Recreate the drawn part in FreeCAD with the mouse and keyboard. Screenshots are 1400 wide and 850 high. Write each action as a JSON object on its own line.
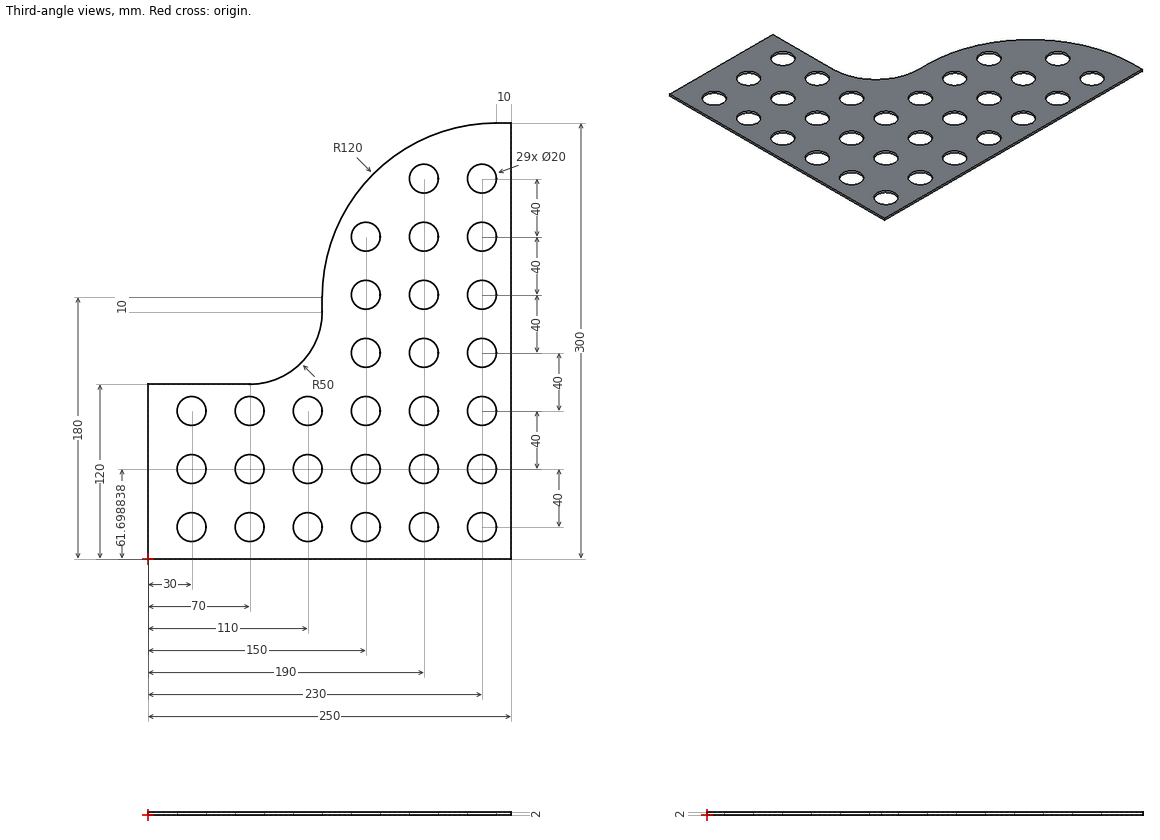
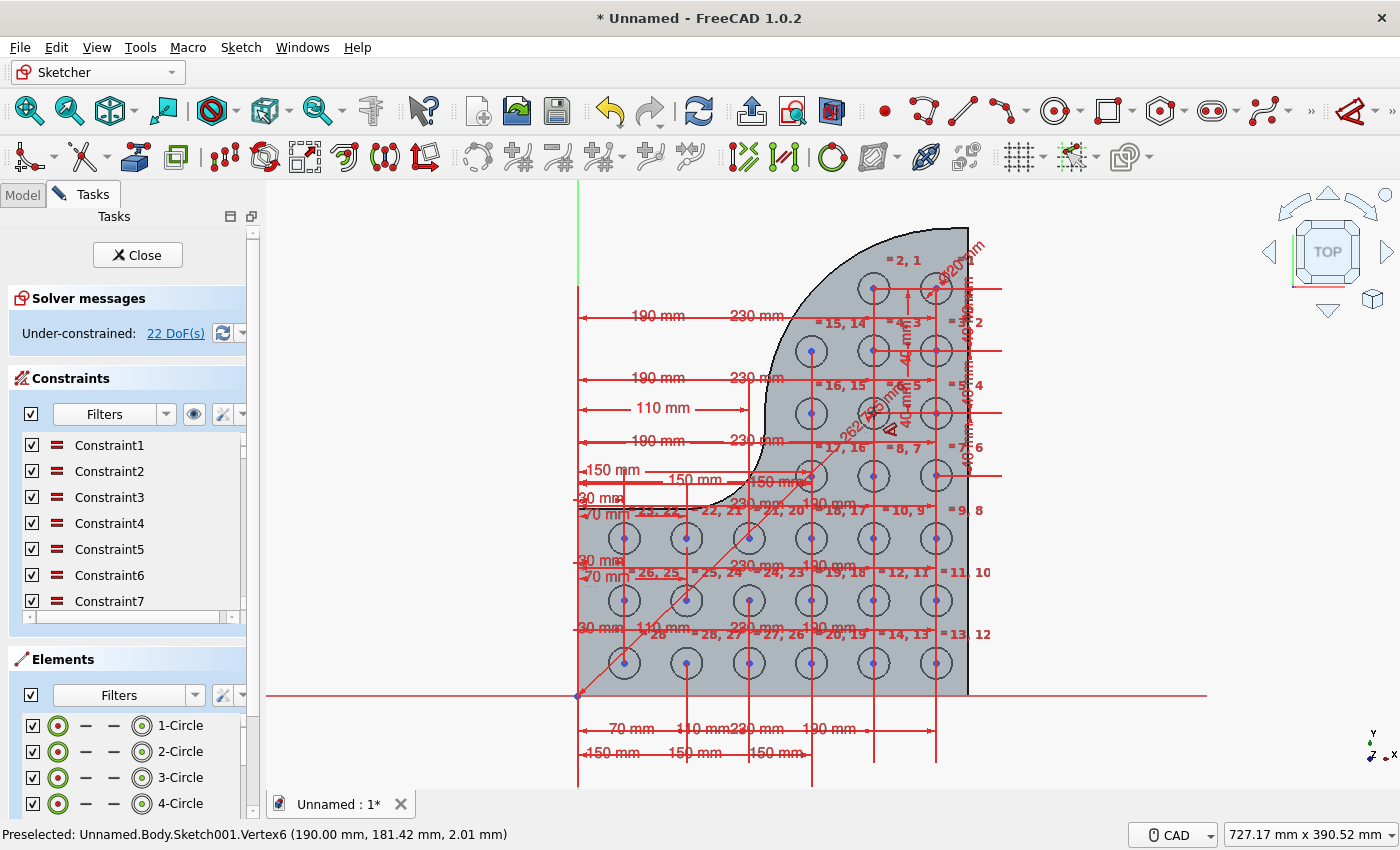
{"action": "left_click", "coordinate": [874, 476]}
{"action": "left_click", "coordinate": [908, 467]}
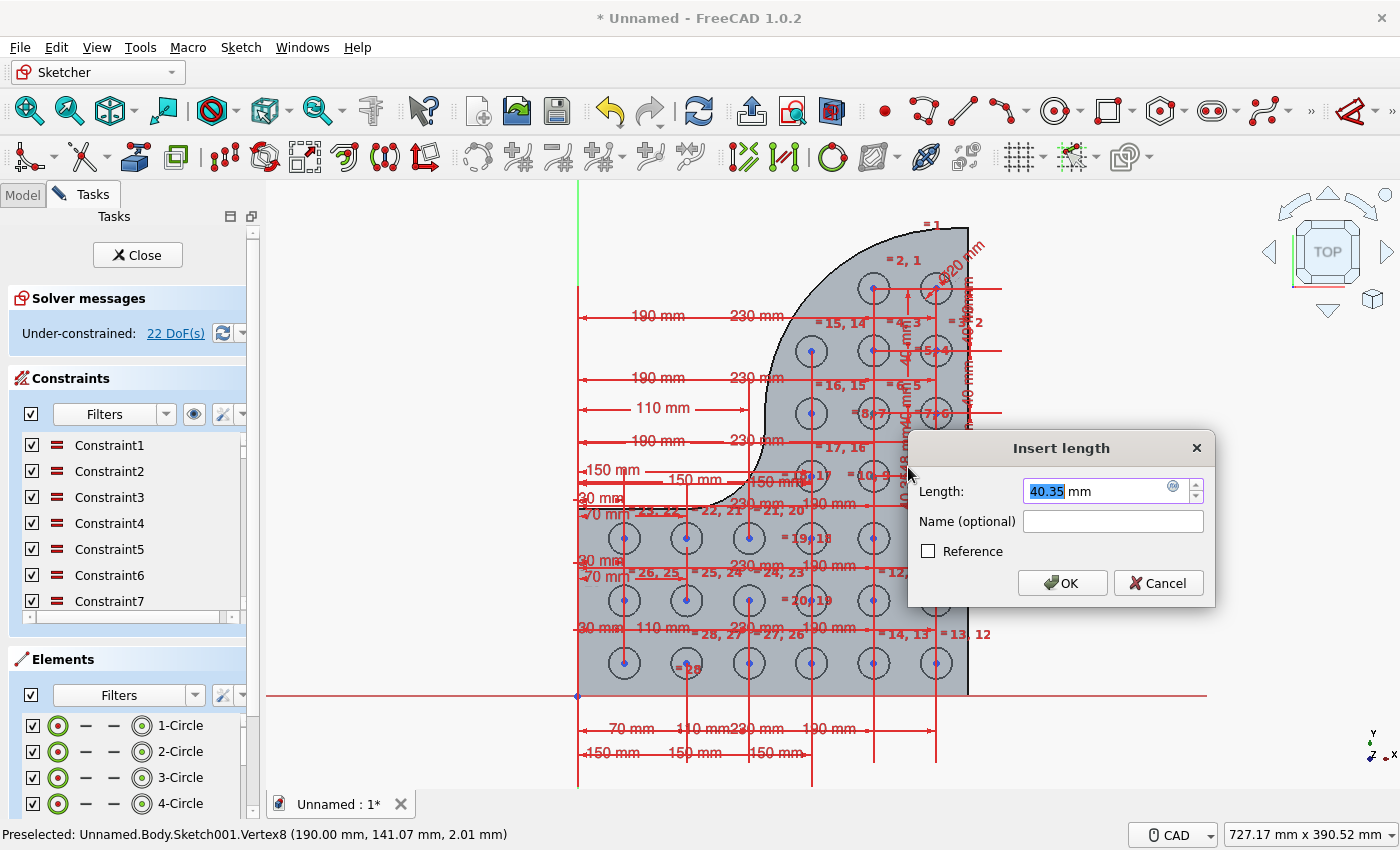
{"action": "type", "text": "40"}
{"action": "key", "text": "Return"}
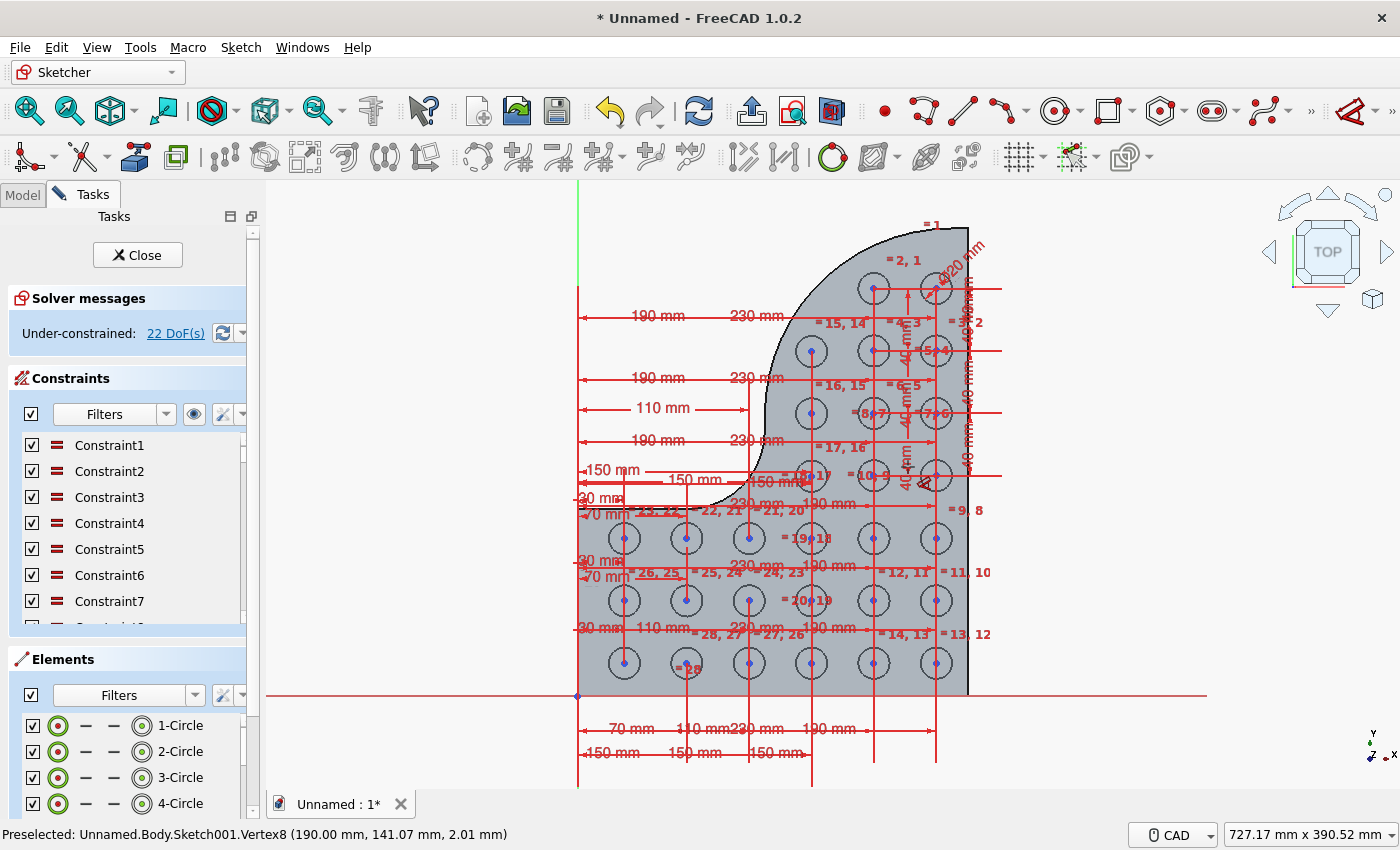
{"action": "left_click", "coordinate": [936, 476]}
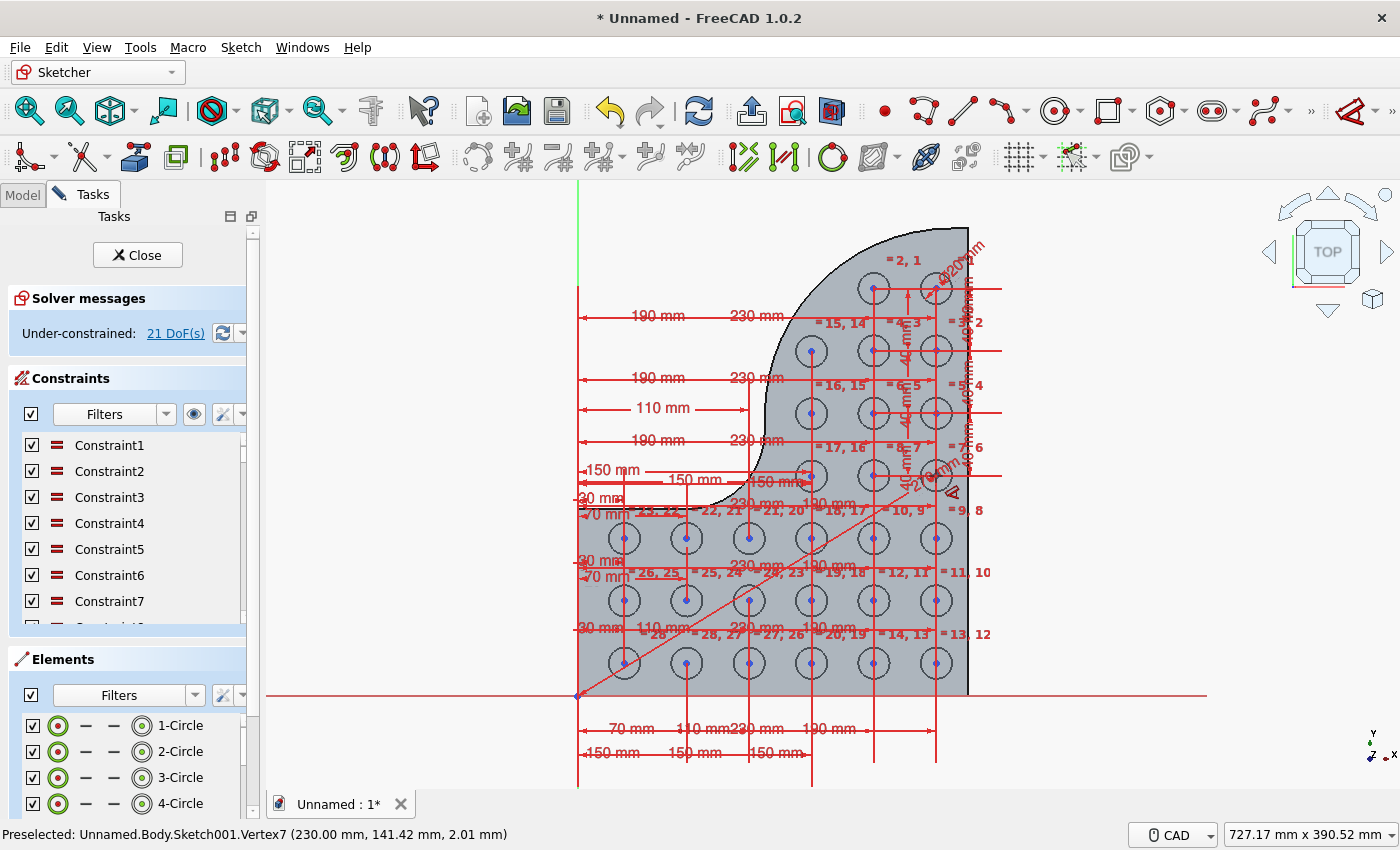
{"action": "left_click", "coordinate": [936, 539]}
{"action": "left_click", "coordinate": [970, 507]}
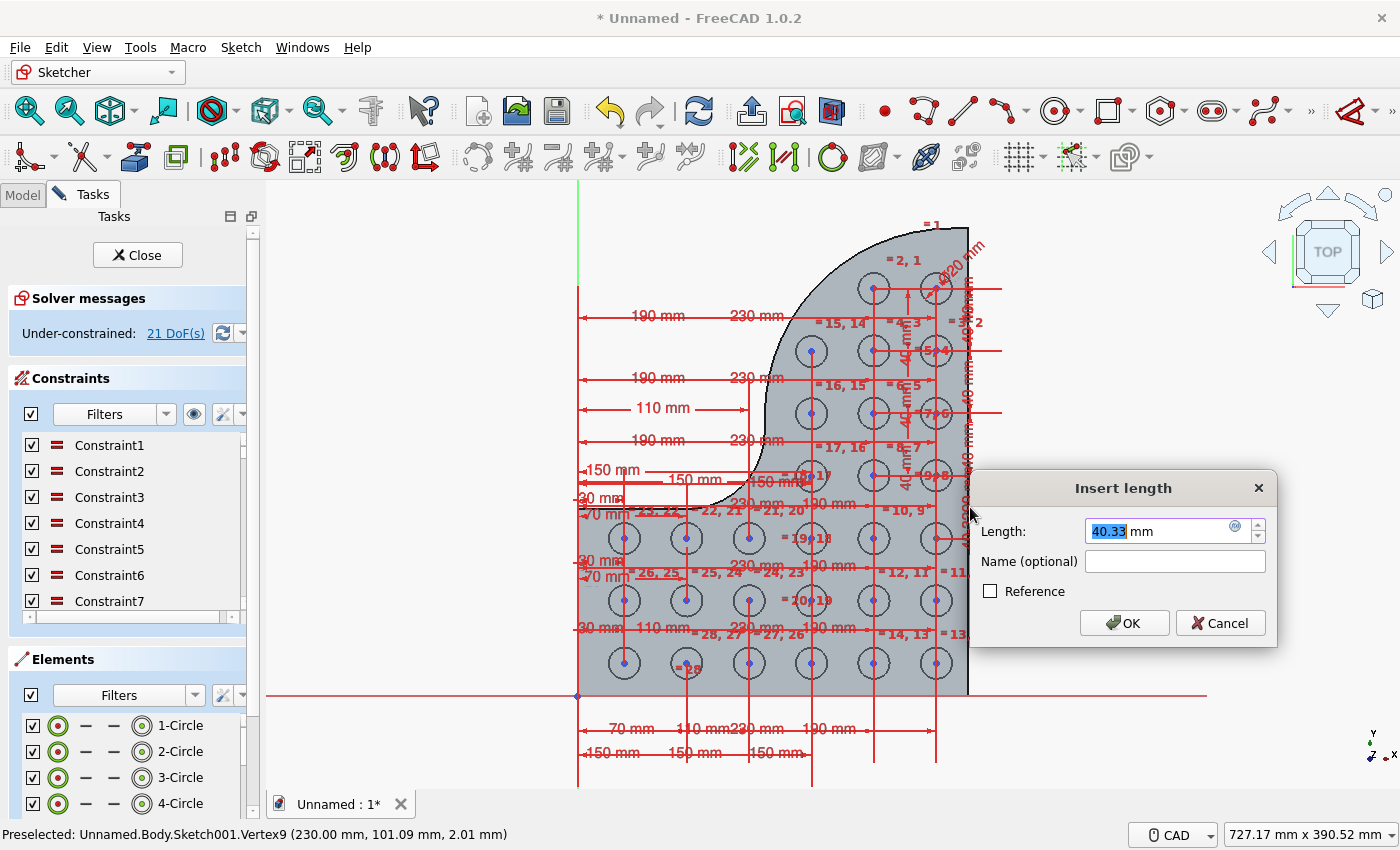
{"action": "type", "text": "40"}
{"action": "key", "text": "Return"}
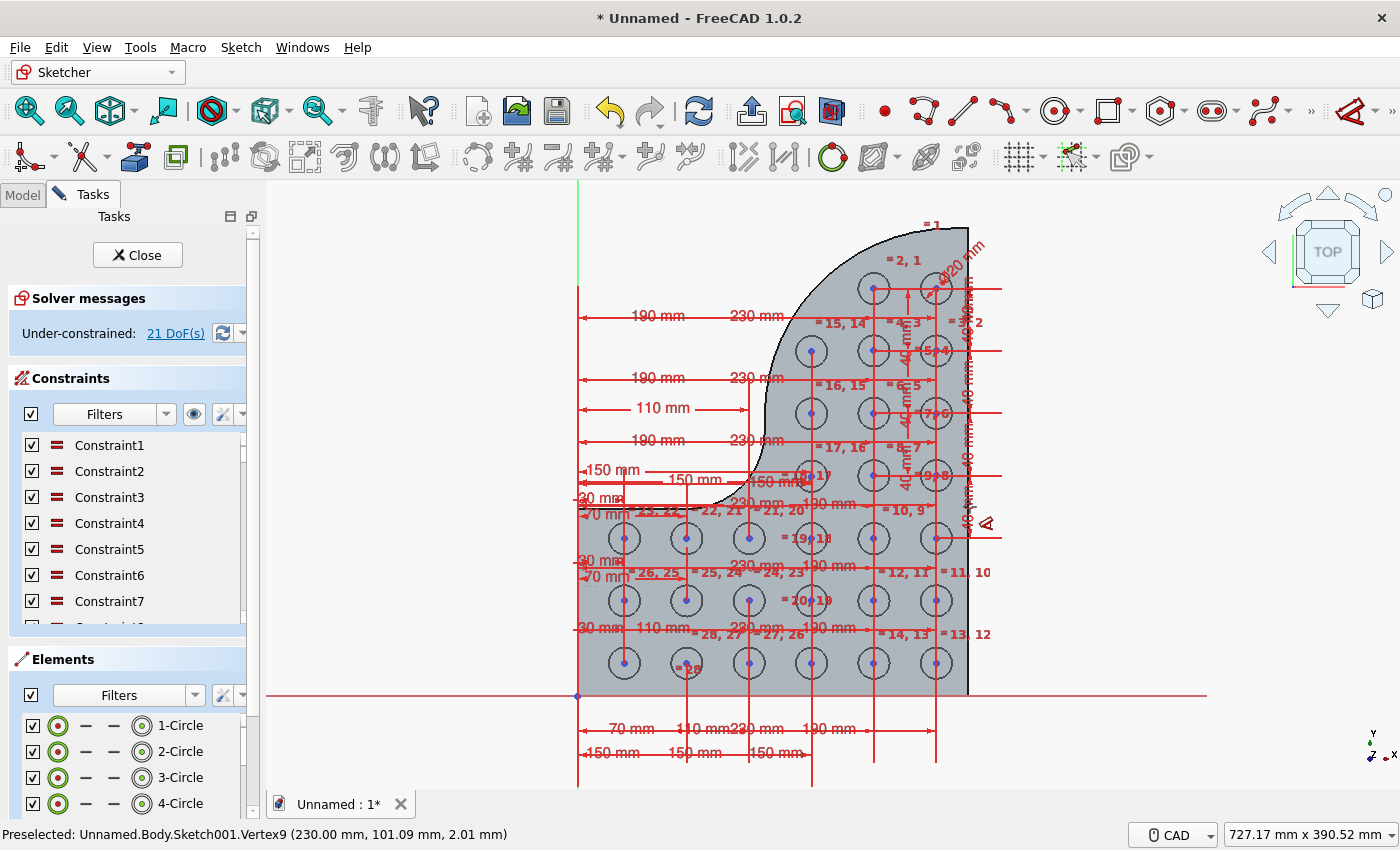
{"action": "left_click", "coordinate": [874, 476]}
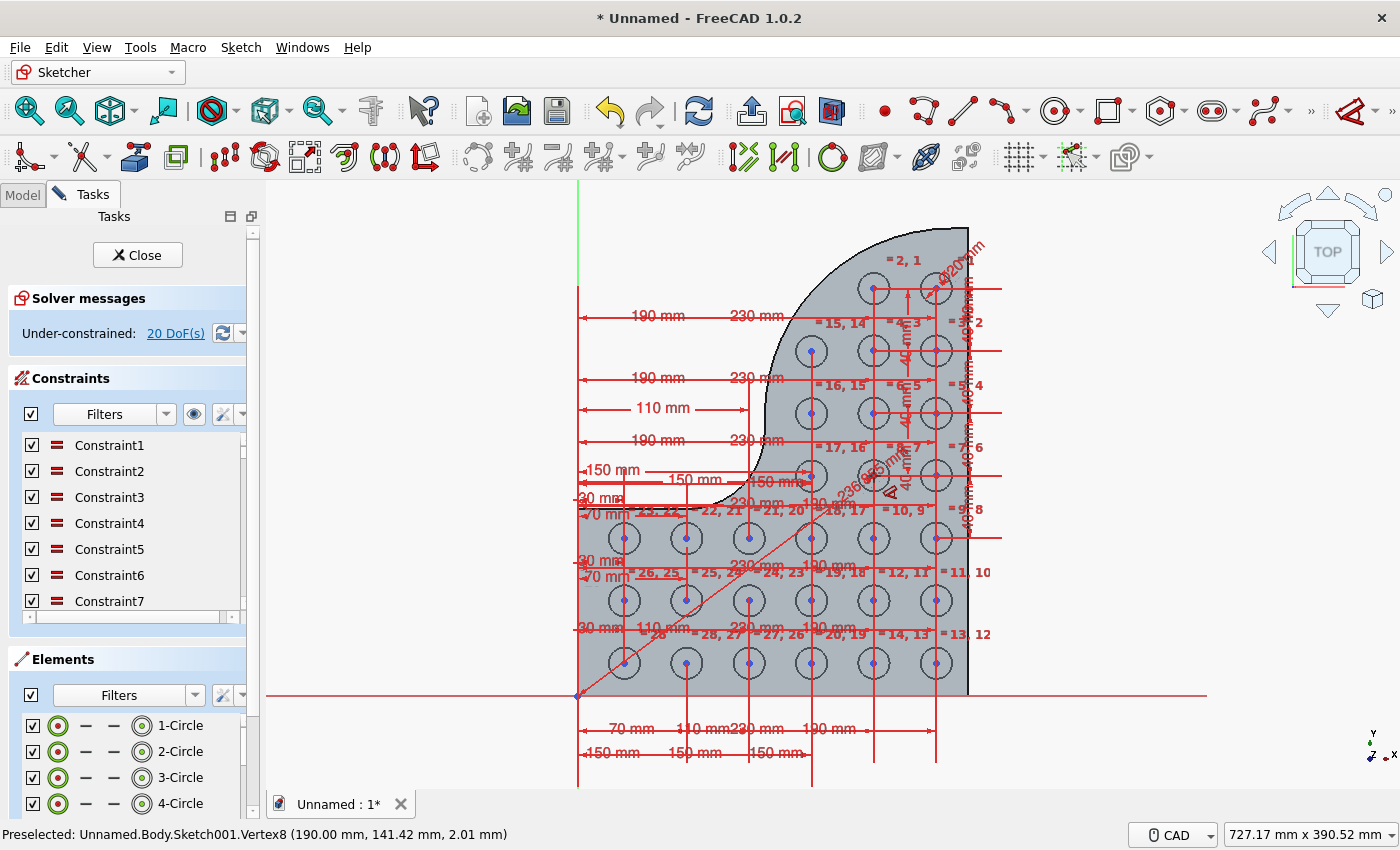
{"action": "left_click", "coordinate": [874, 539]}
{"action": "left_click", "coordinate": [908, 529]}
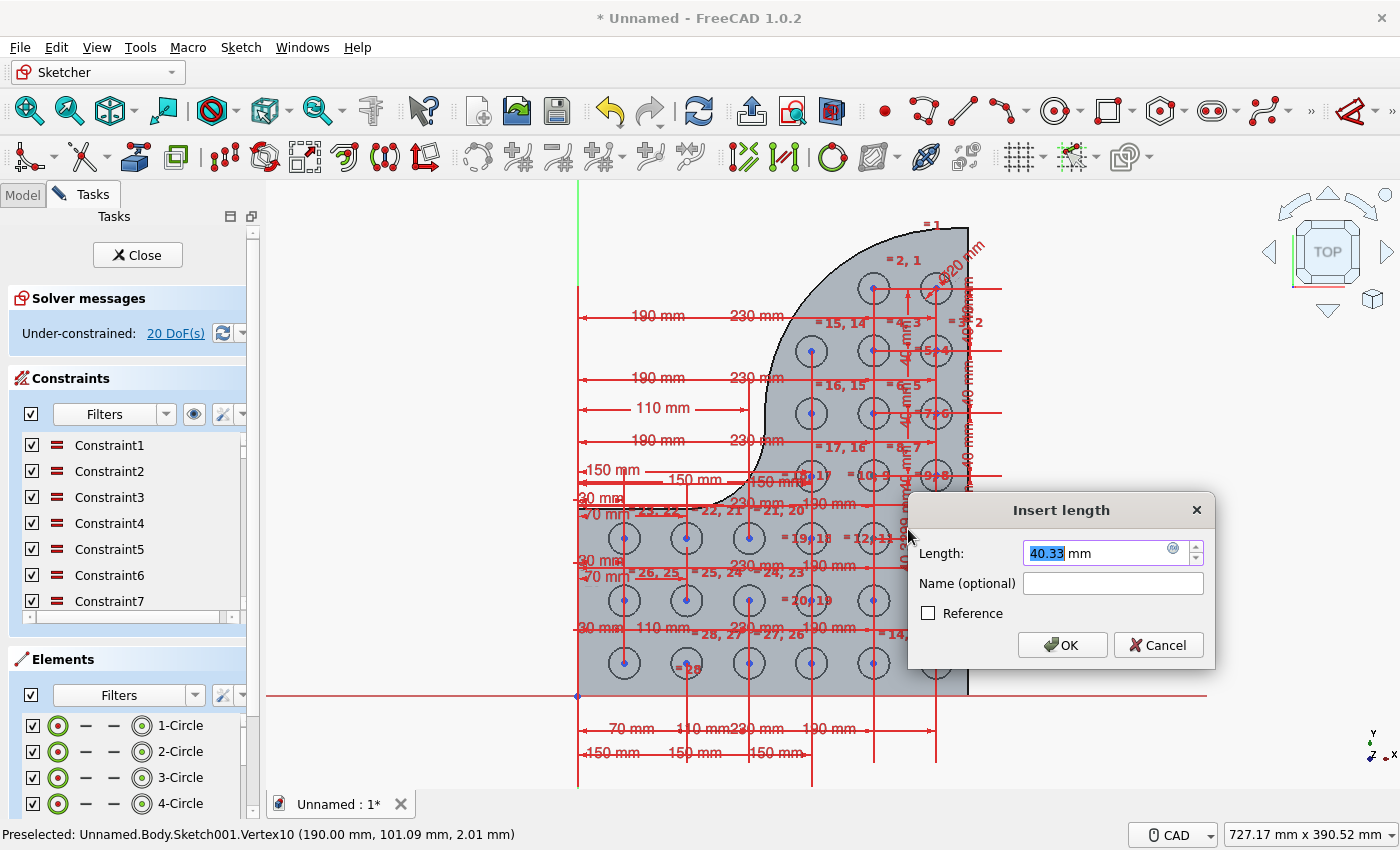
{"action": "type", "text": "40"}
{"action": "key", "text": "Return"}